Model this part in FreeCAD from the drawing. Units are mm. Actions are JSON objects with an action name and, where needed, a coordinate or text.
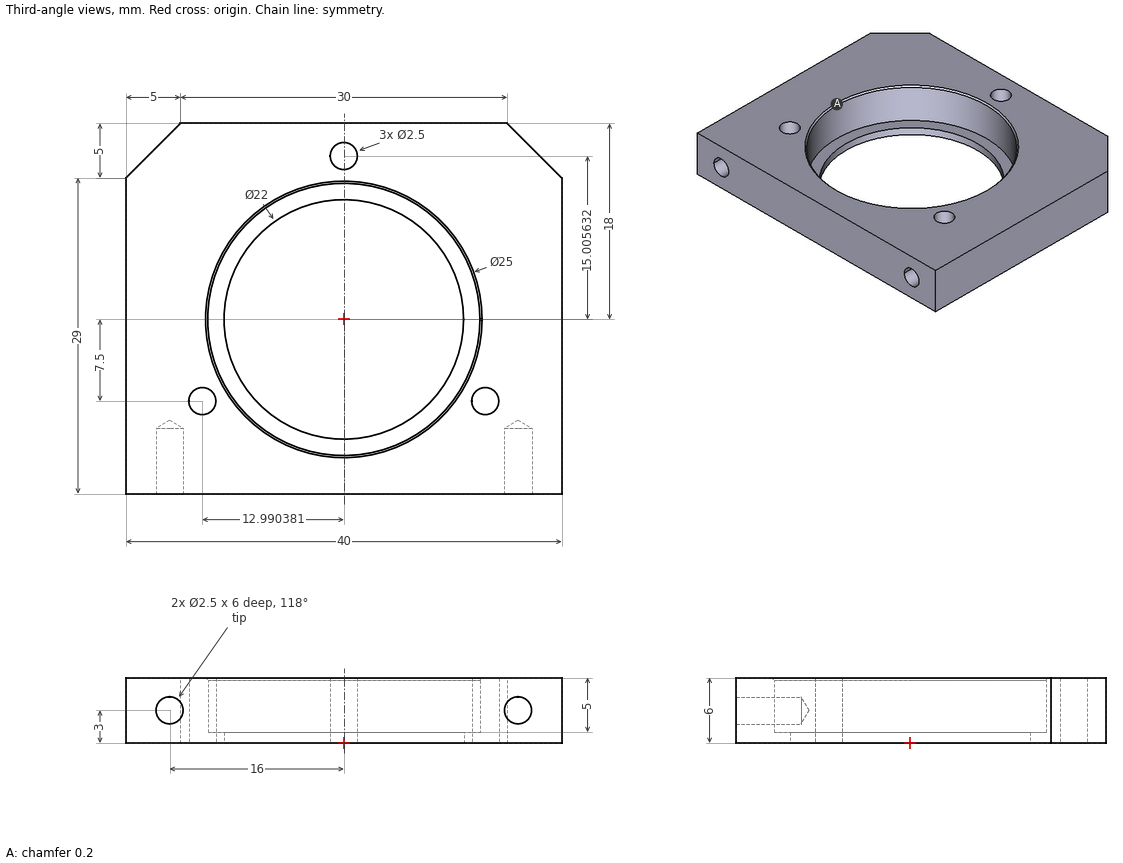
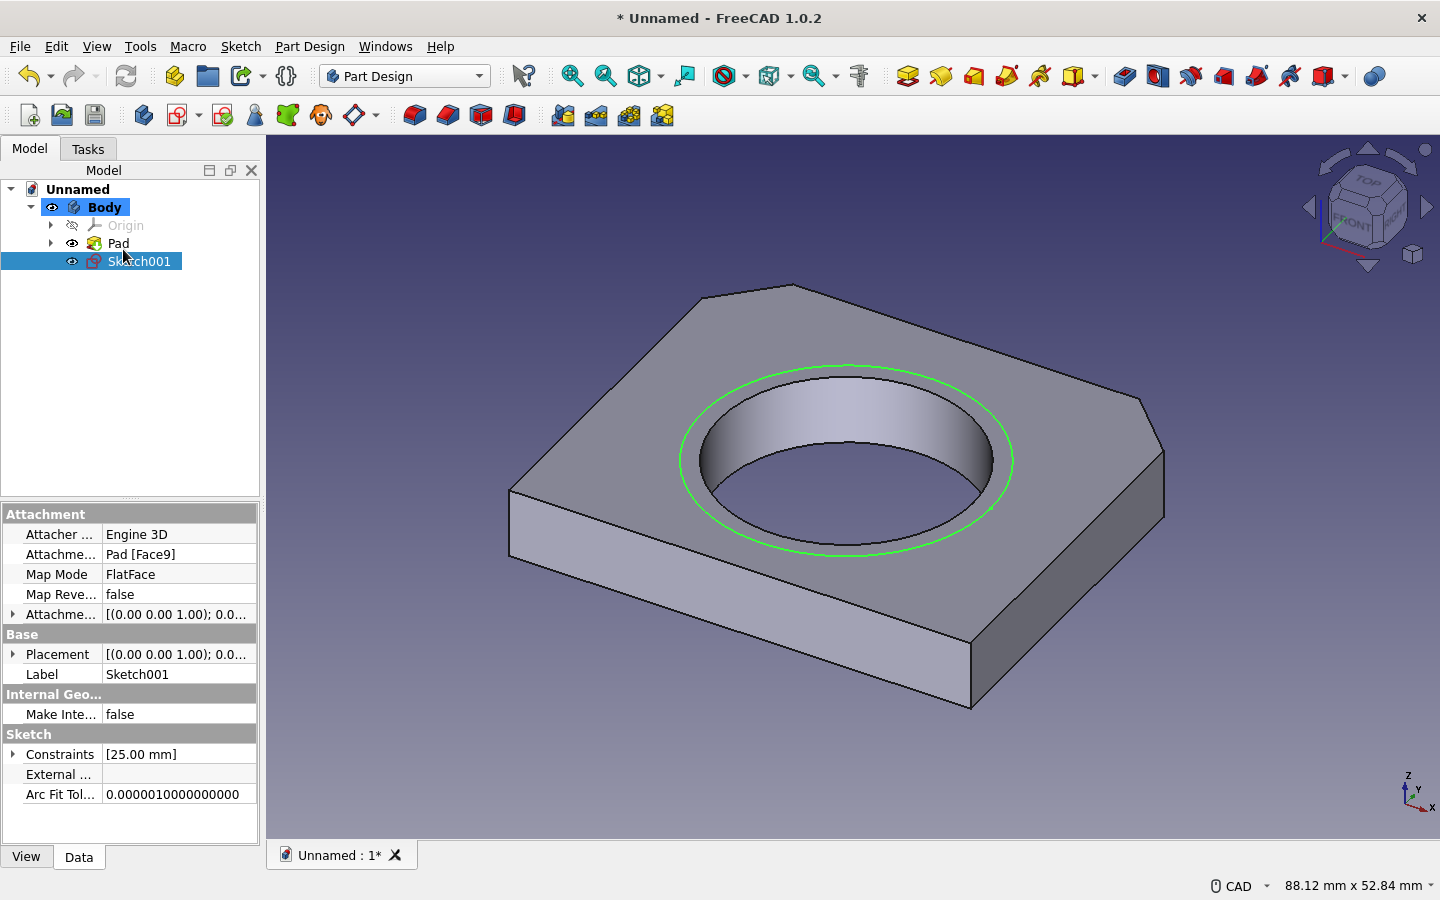
{"action": "left_click", "coordinate": [1125, 76]}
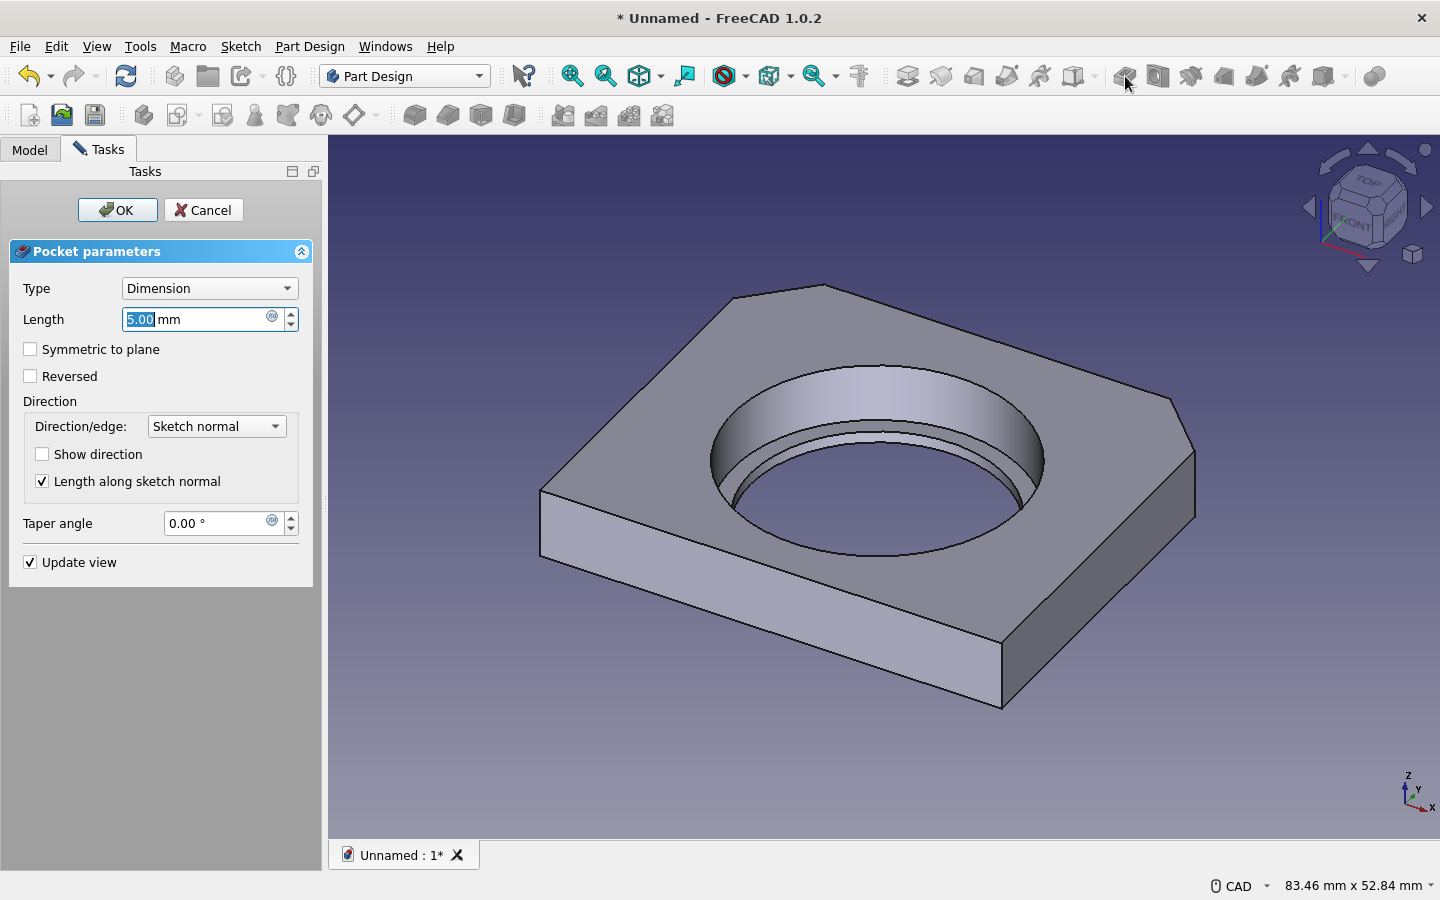
{"action": "type", "text": "5"}
{"action": "key", "text": "Tab"}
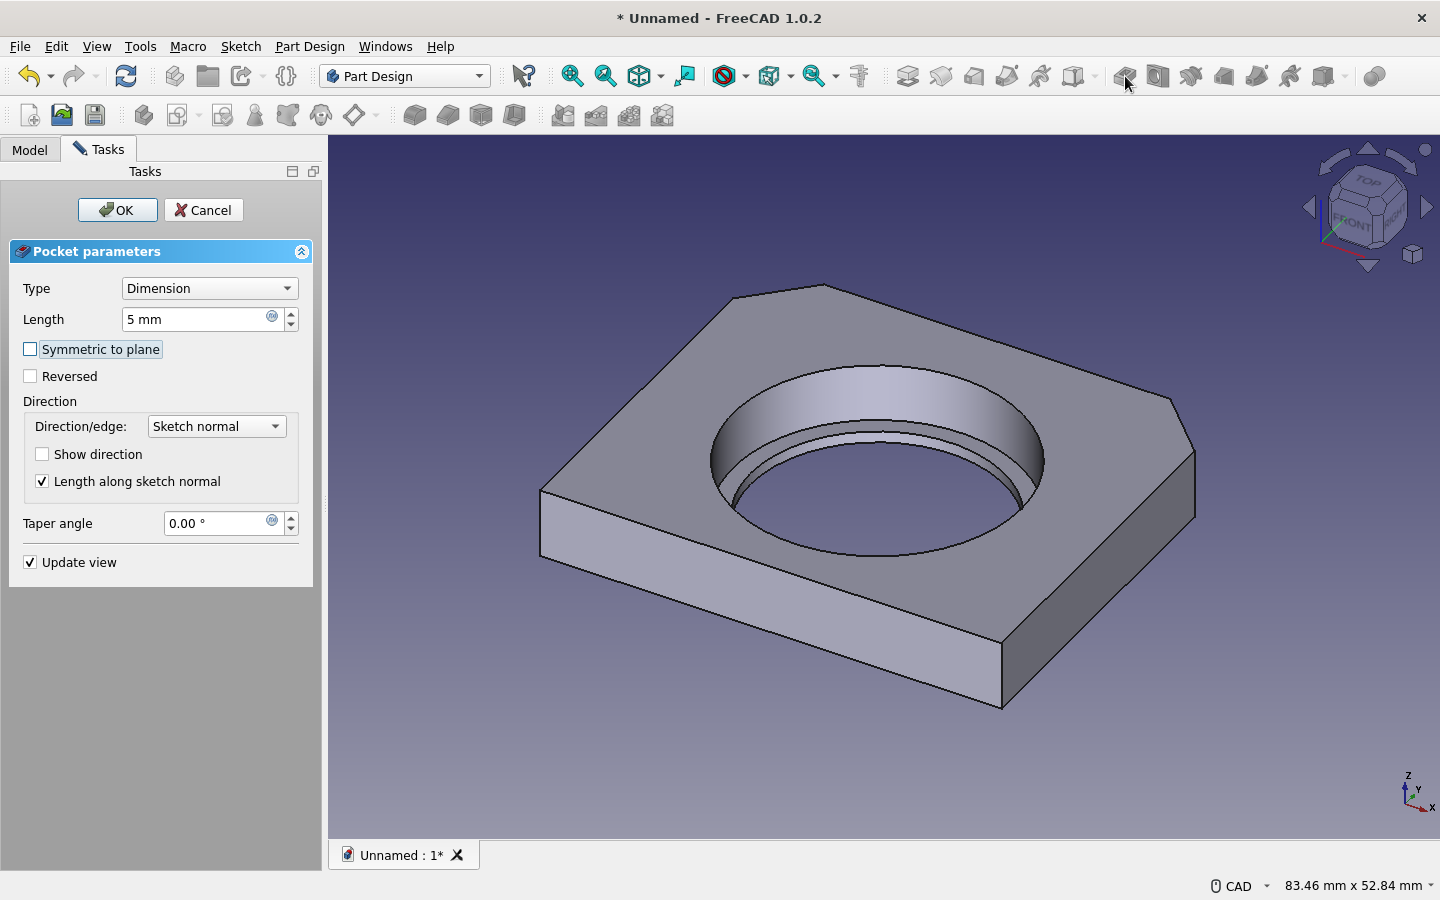
{"action": "left_click", "coordinate": [118, 210]}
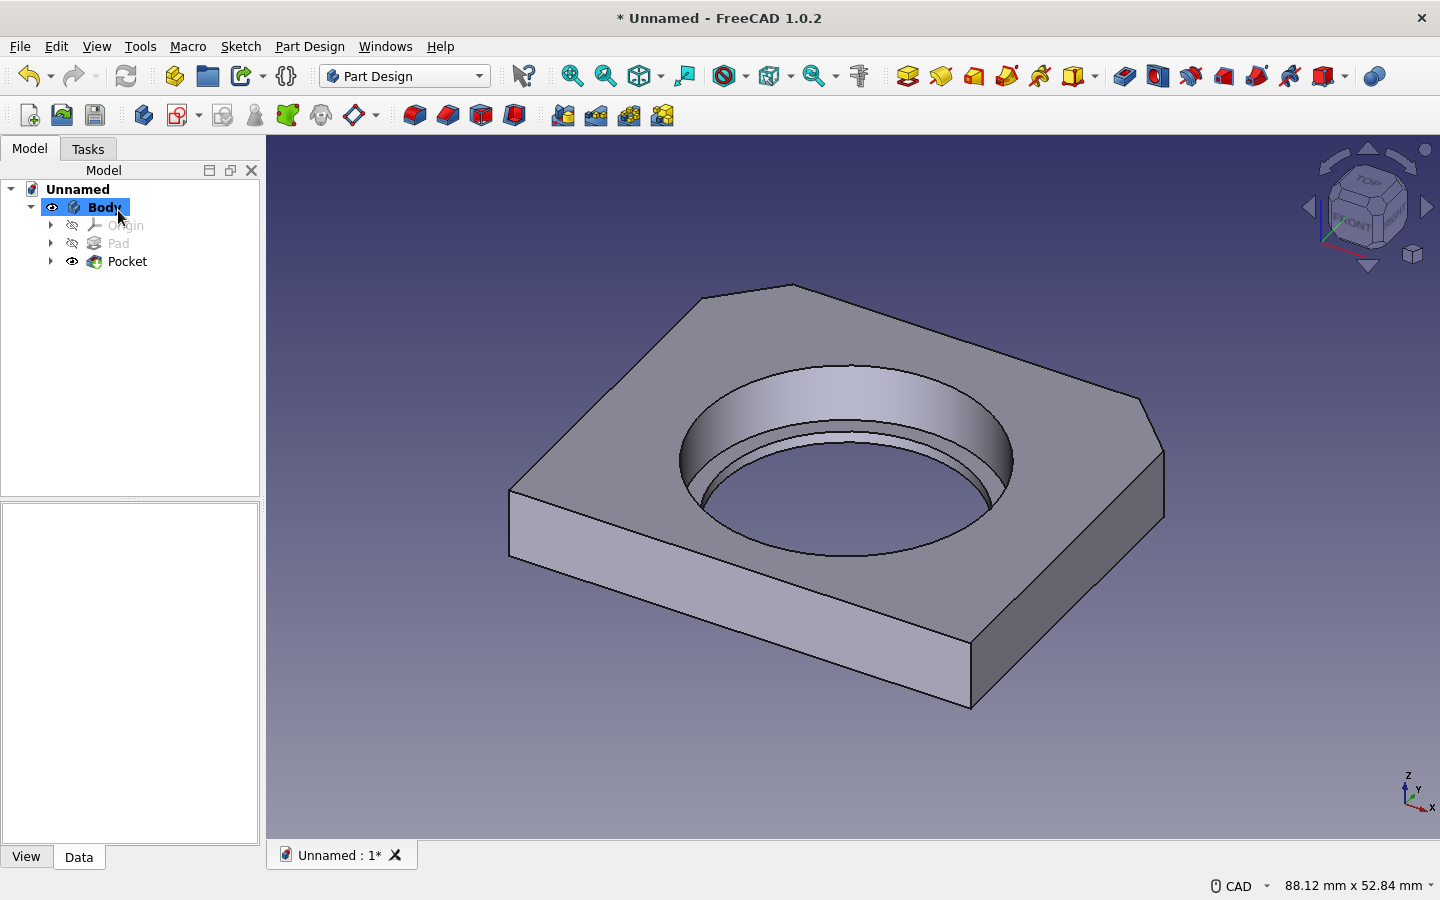
{"action": "left_click", "coordinate": [786, 345]}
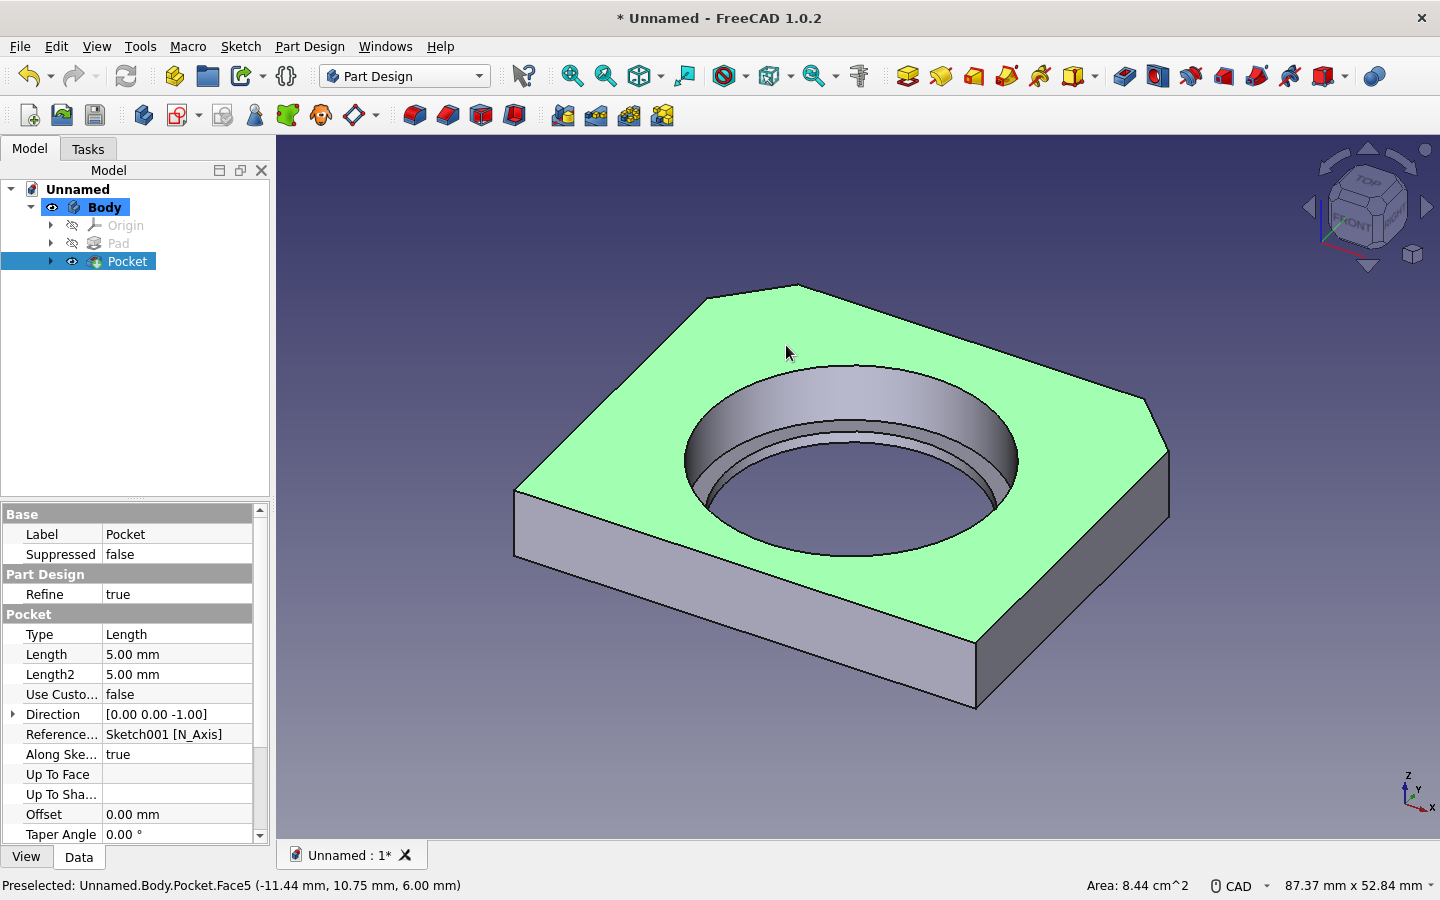
{"action": "left_click", "coordinate": [176, 116]}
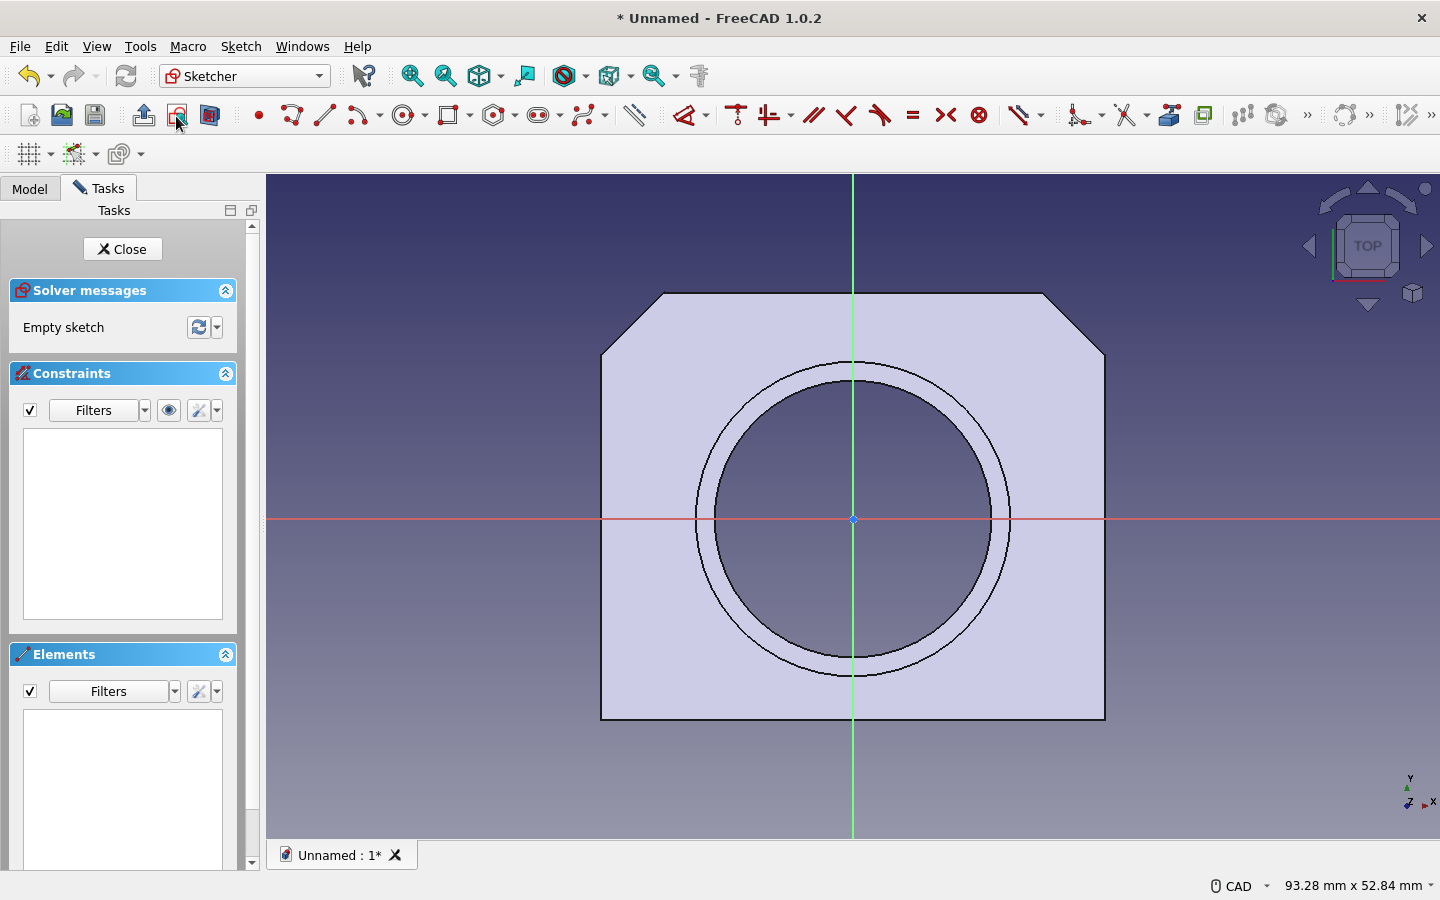
{"action": "scroll", "coordinate": [992, 401], "scroll_direction": "up", "scroll_amount": 2}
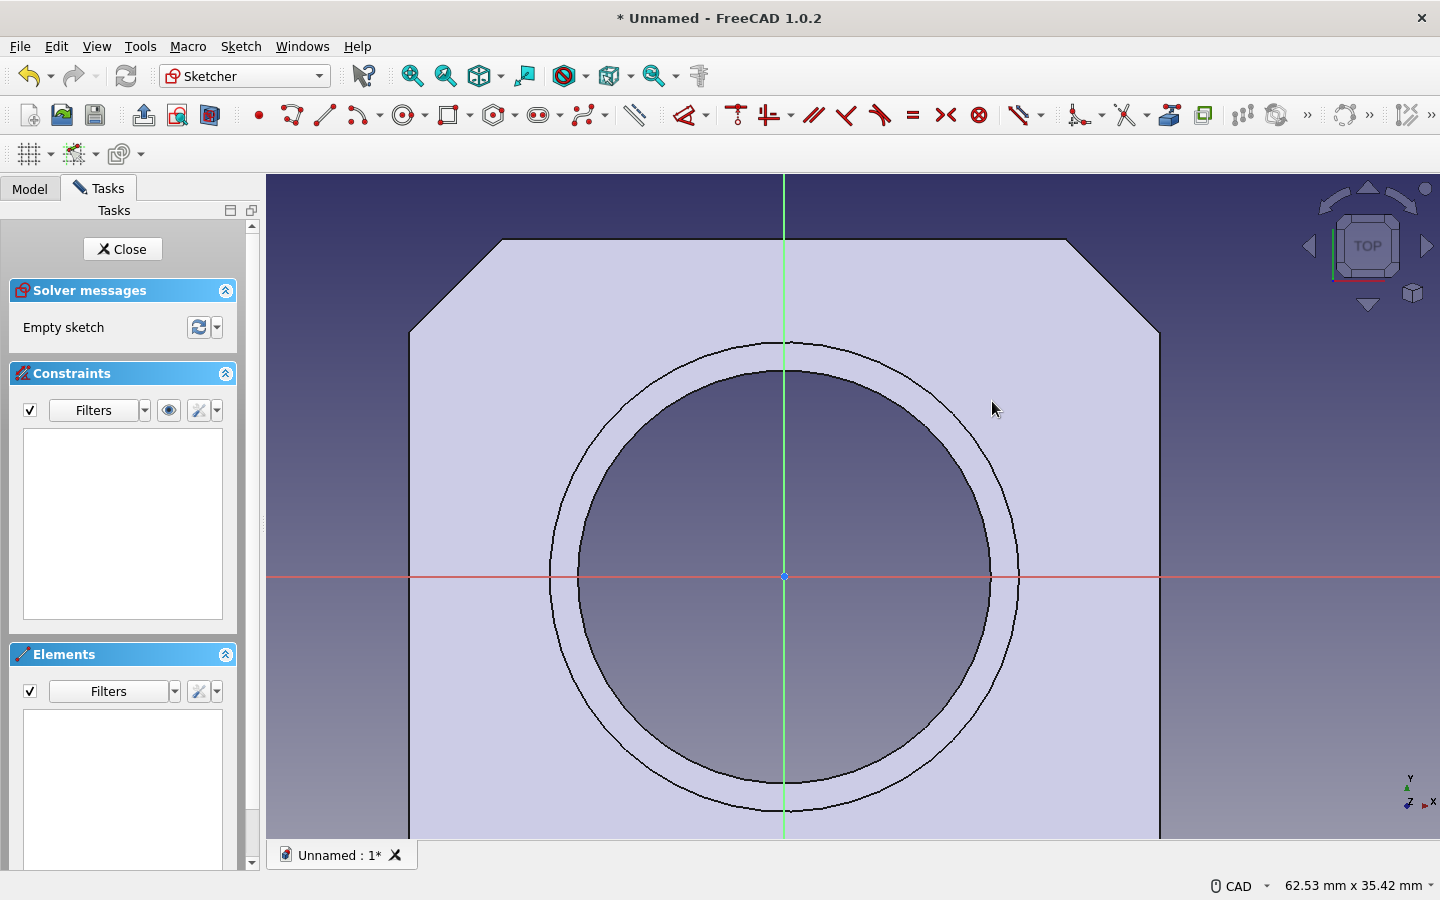
{"action": "left_click", "coordinate": [402, 116]}